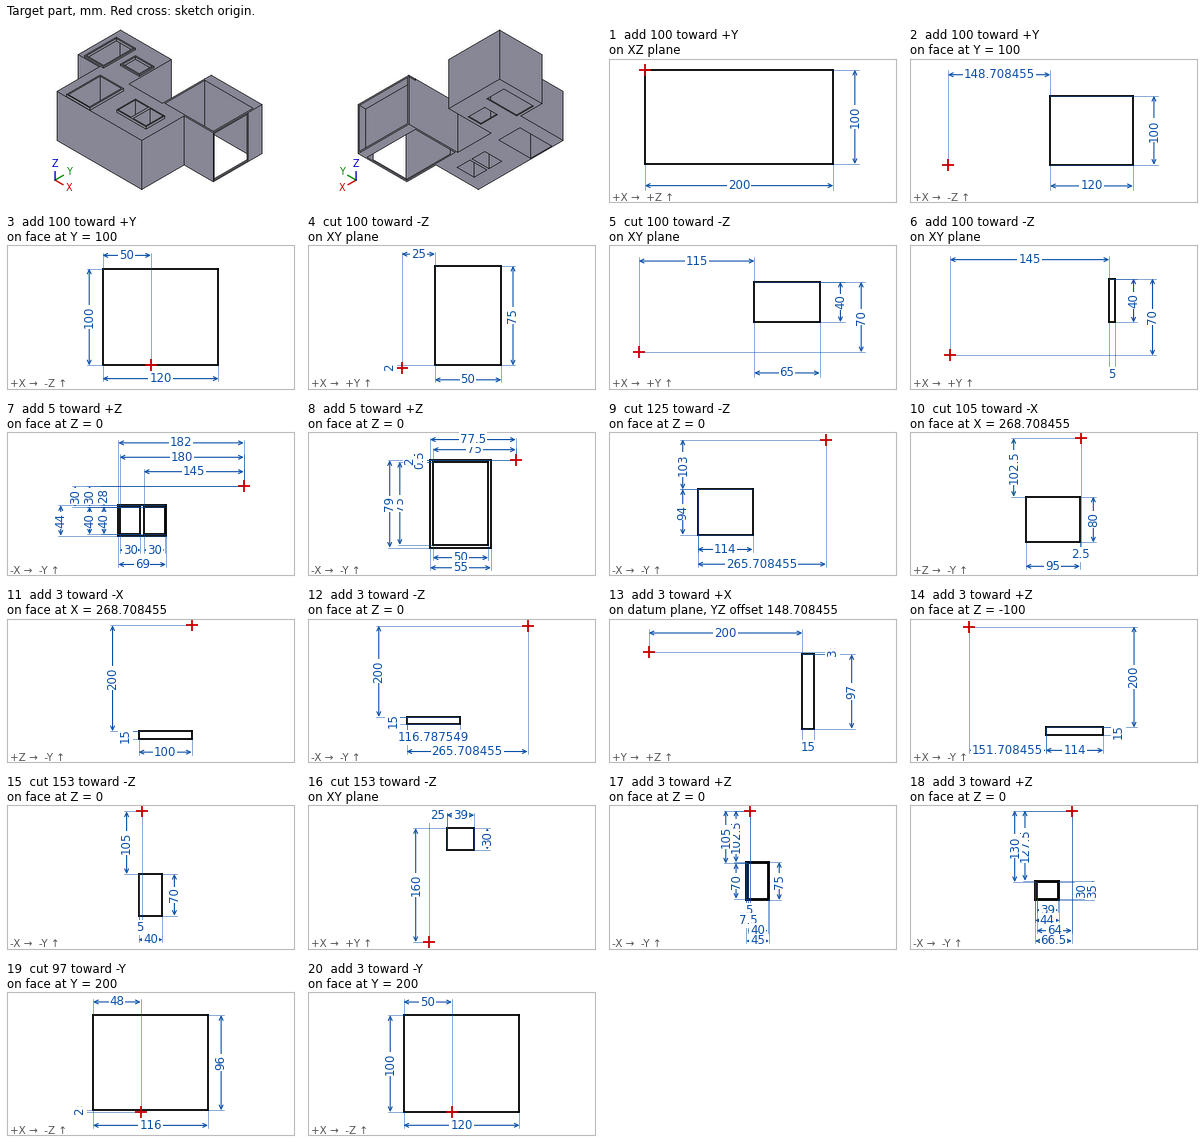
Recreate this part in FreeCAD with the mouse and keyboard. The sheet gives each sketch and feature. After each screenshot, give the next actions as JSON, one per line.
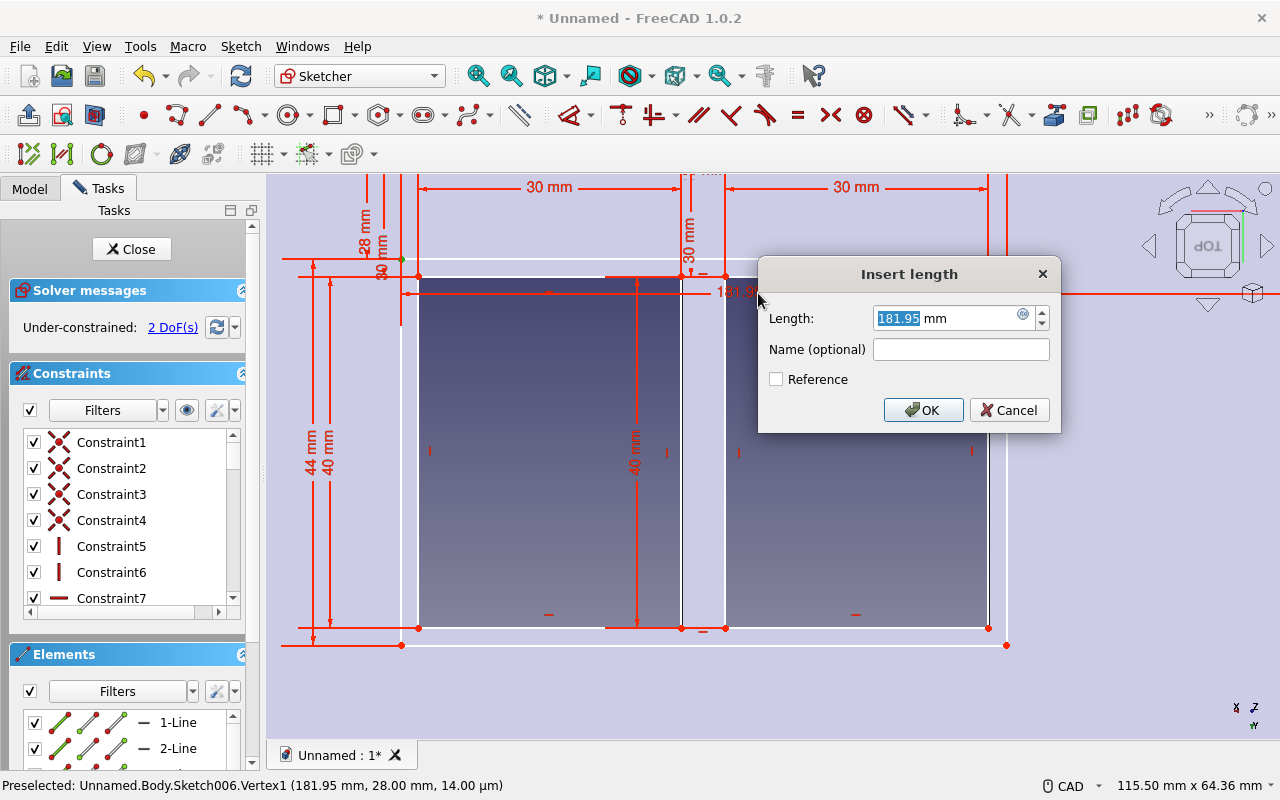
{"action": "type", "text": "182"}
{"action": "key", "text": "Return"}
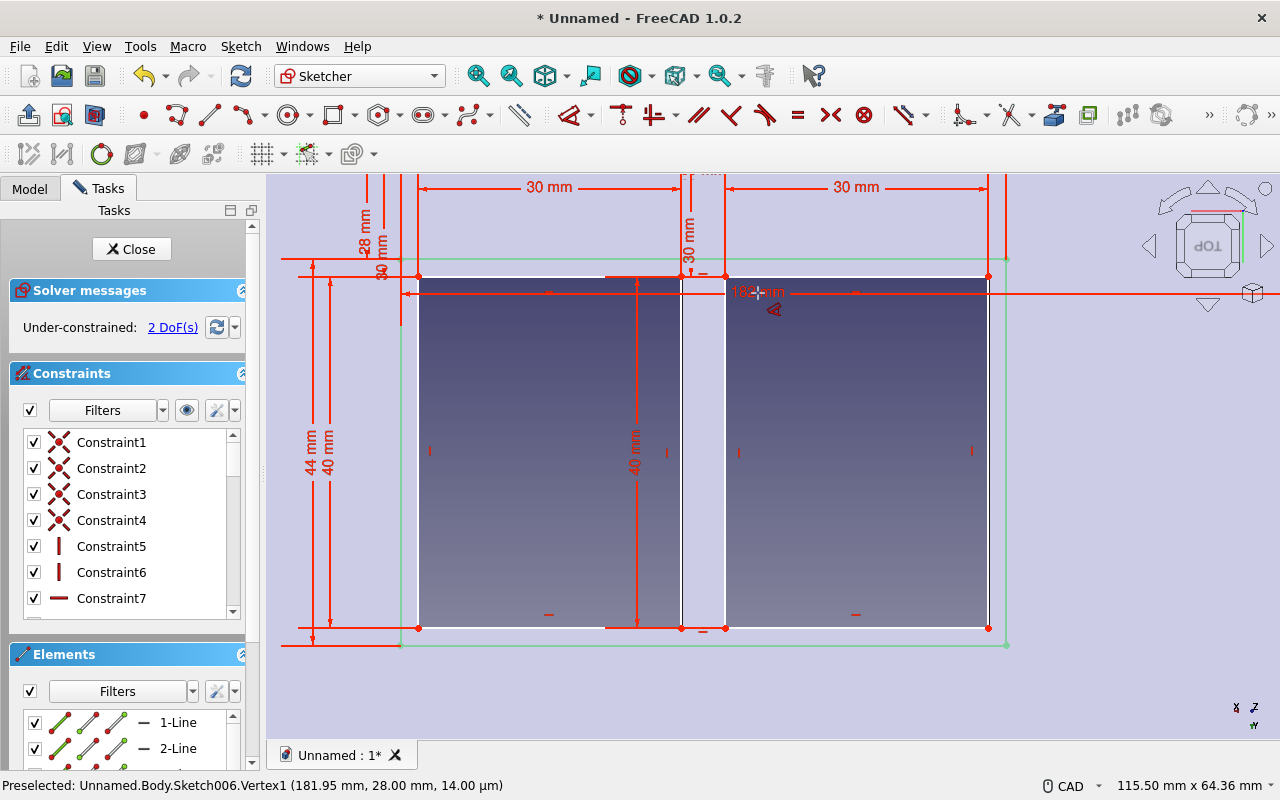
{"action": "left_click", "coordinate": [725, 277]}
{"action": "left_click", "coordinate": [920, 311]}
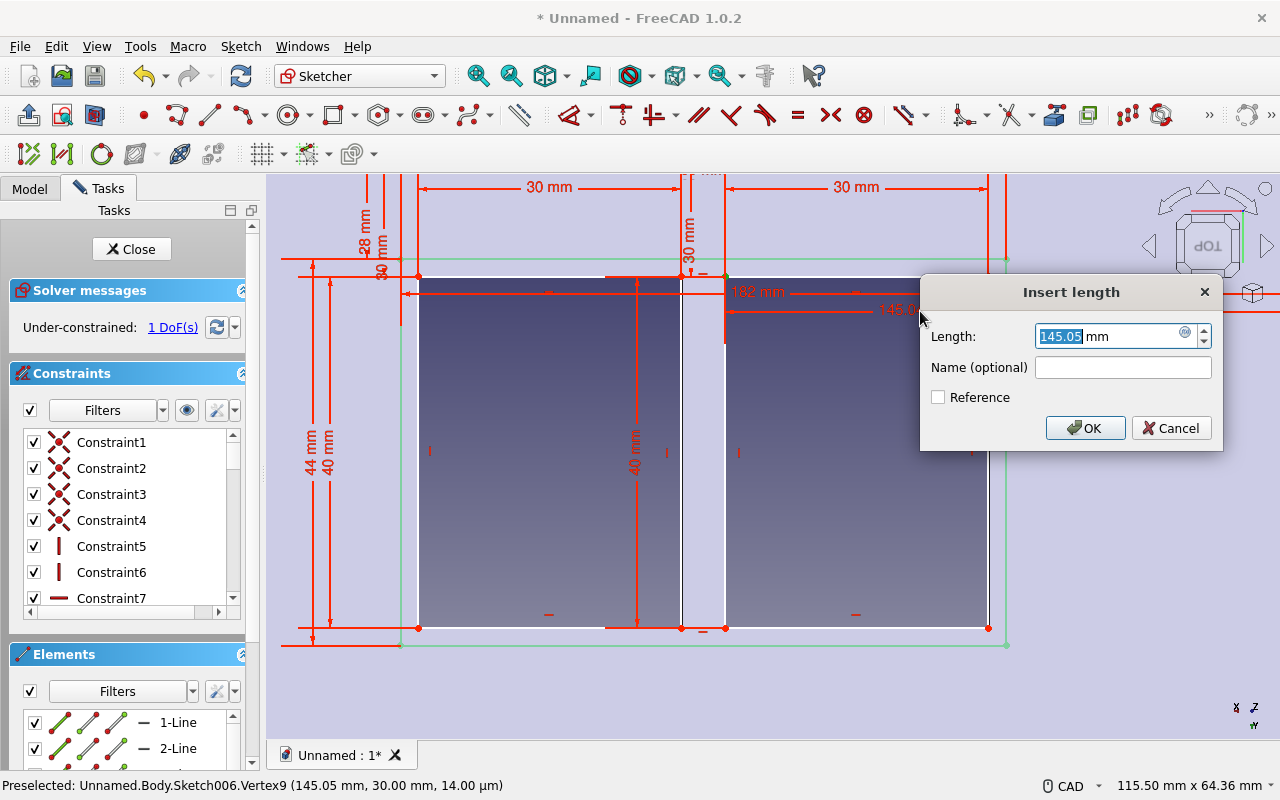
{"action": "type", "text": "145"}
{"action": "key", "text": "Return"}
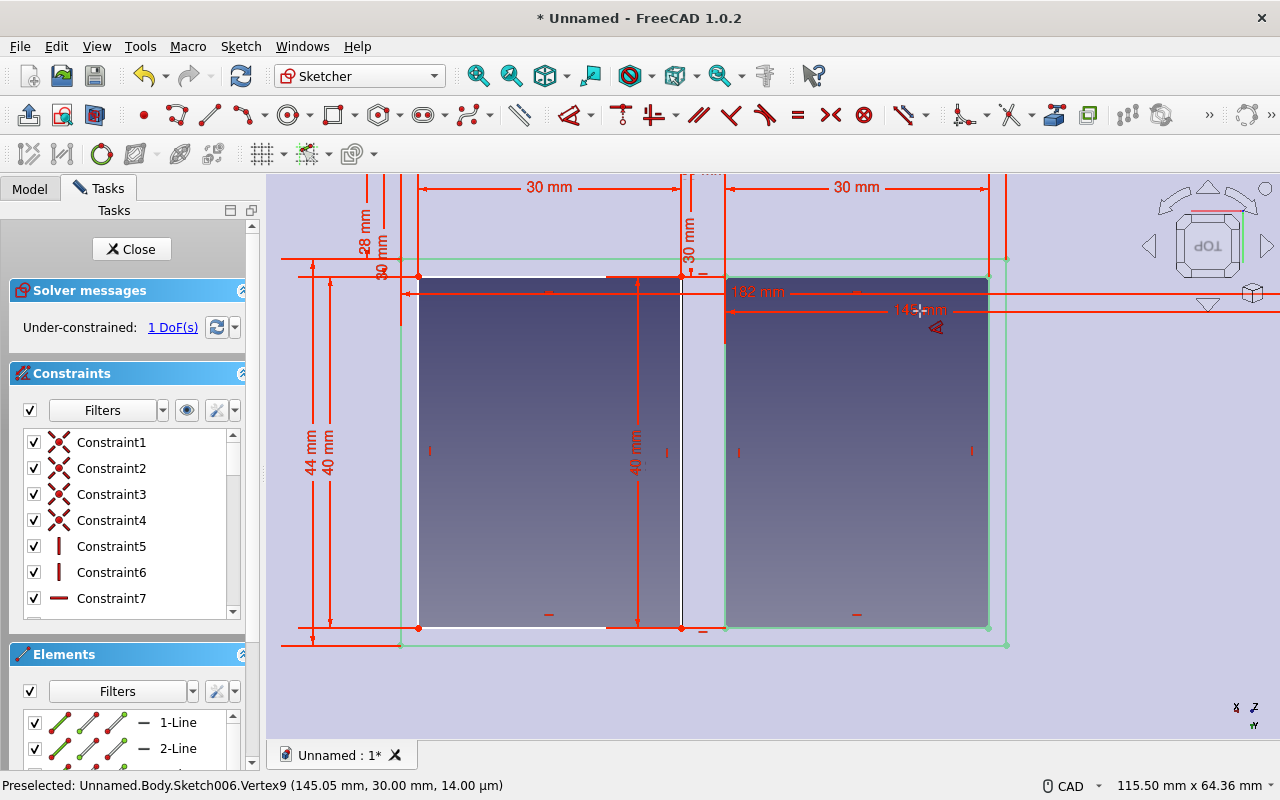
{"action": "left_click", "coordinate": [418, 277]}
{"action": "left_click", "coordinate": [606, 311]}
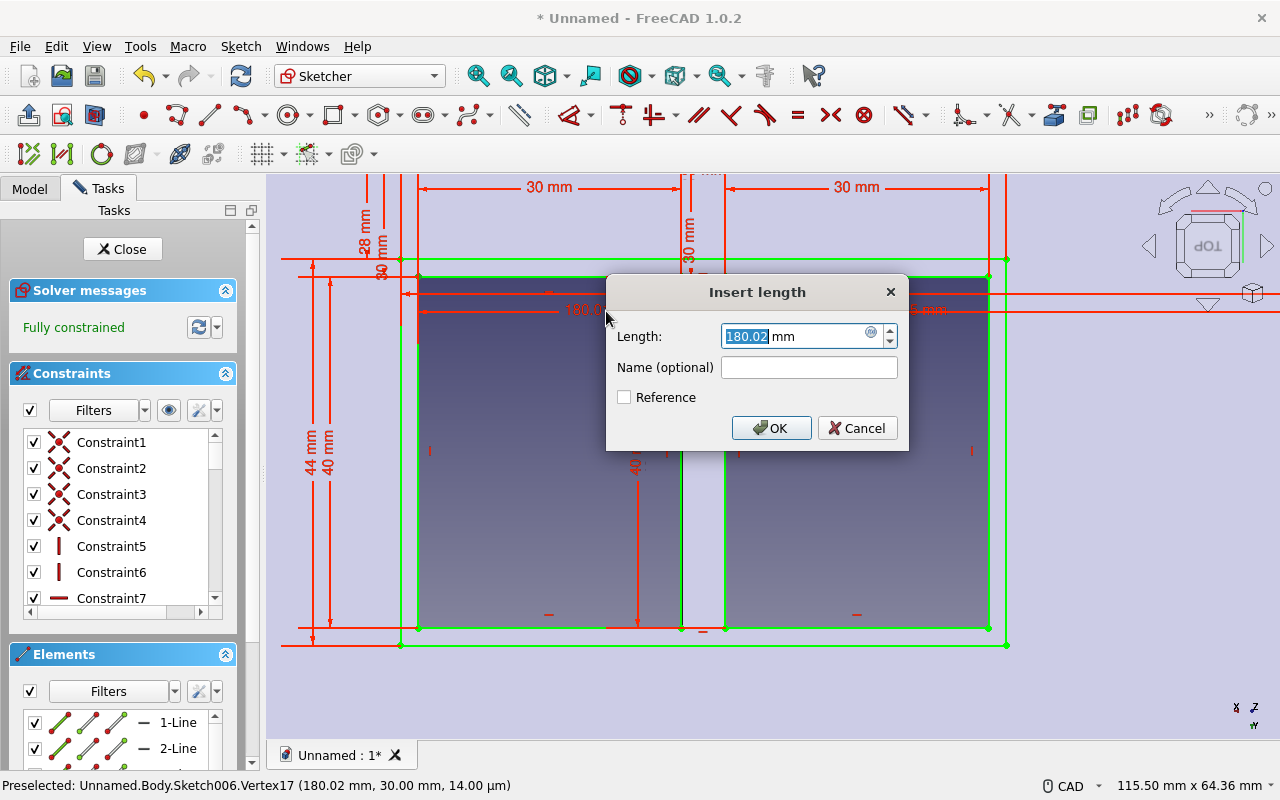
{"action": "type", "text": "180"}
{"action": "key", "text": "Return"}
{"action": "key", "text": "Escape"}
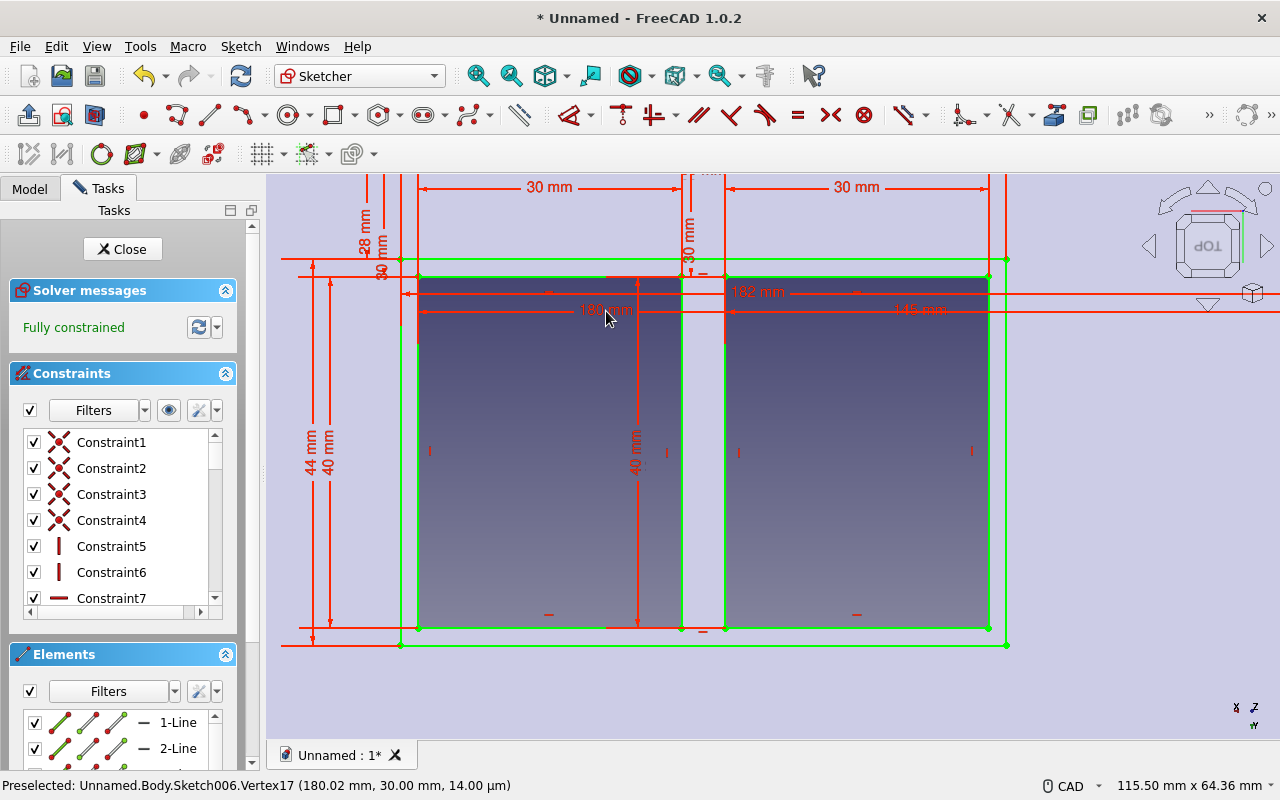
{"action": "left_click", "coordinate": [123, 249]}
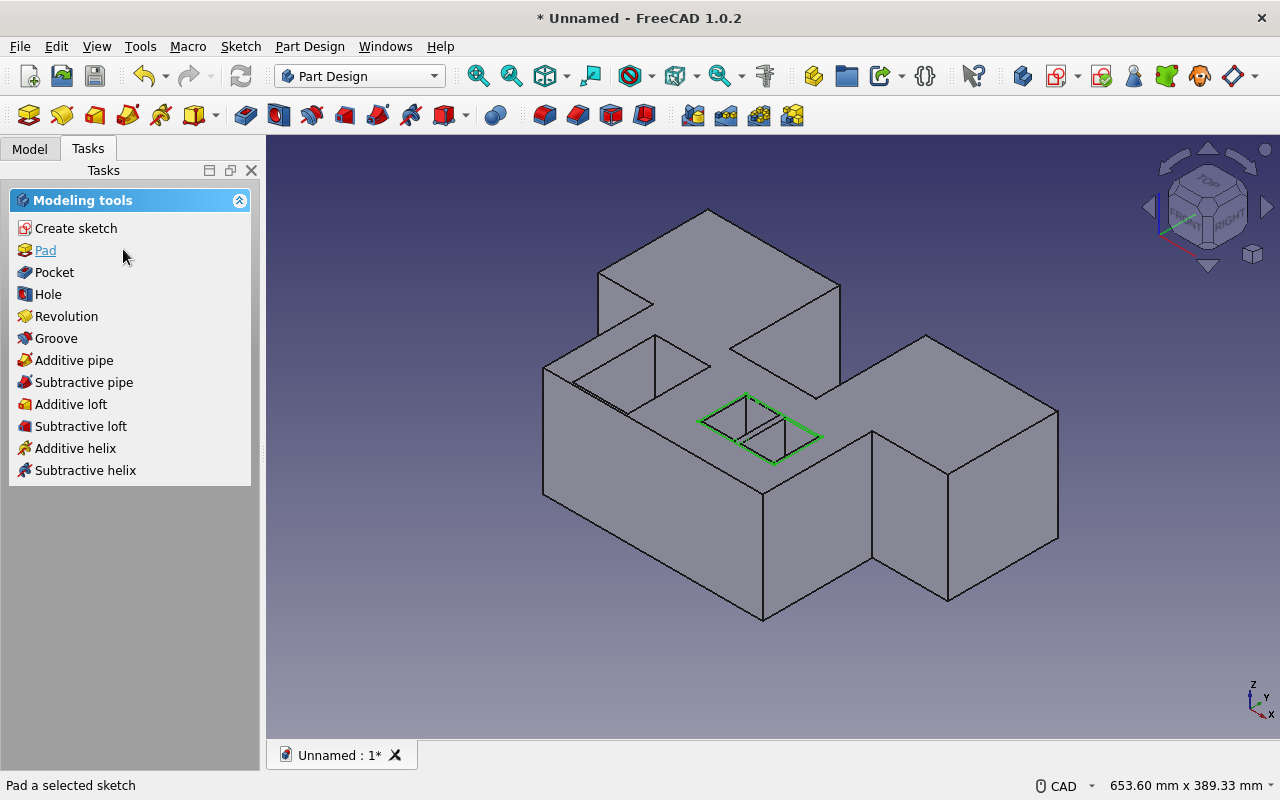
{"action": "left_click", "coordinate": [29, 116]}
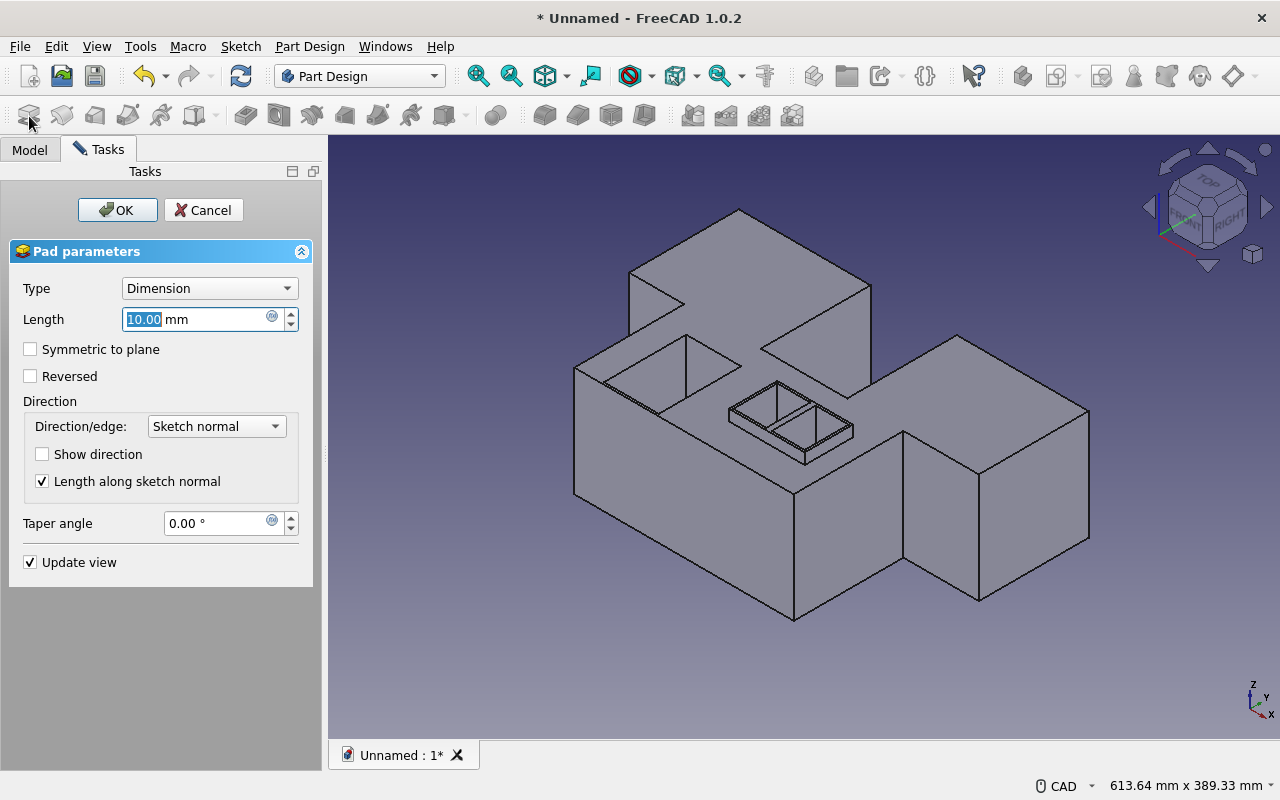
{"action": "type", "text": "5"}
{"action": "key", "text": "Tab"}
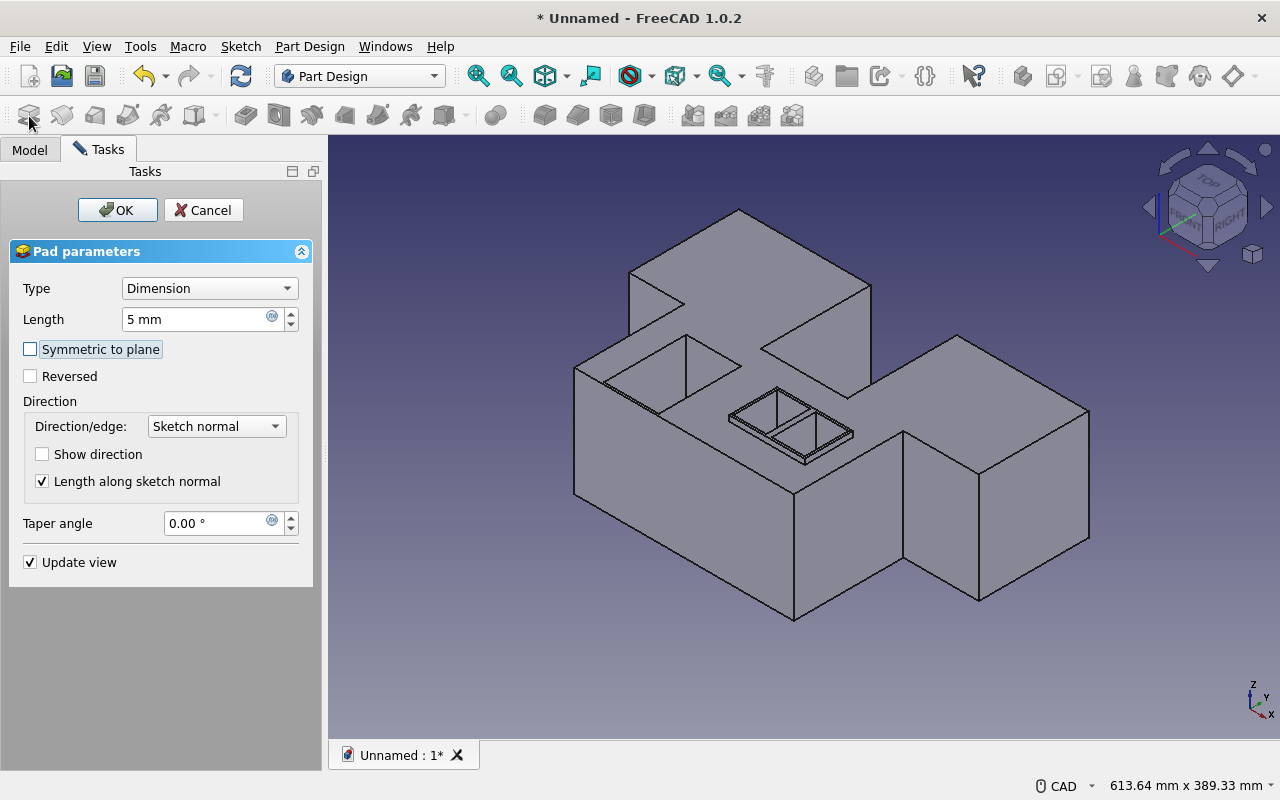
{"action": "left_click", "coordinate": [118, 210]}